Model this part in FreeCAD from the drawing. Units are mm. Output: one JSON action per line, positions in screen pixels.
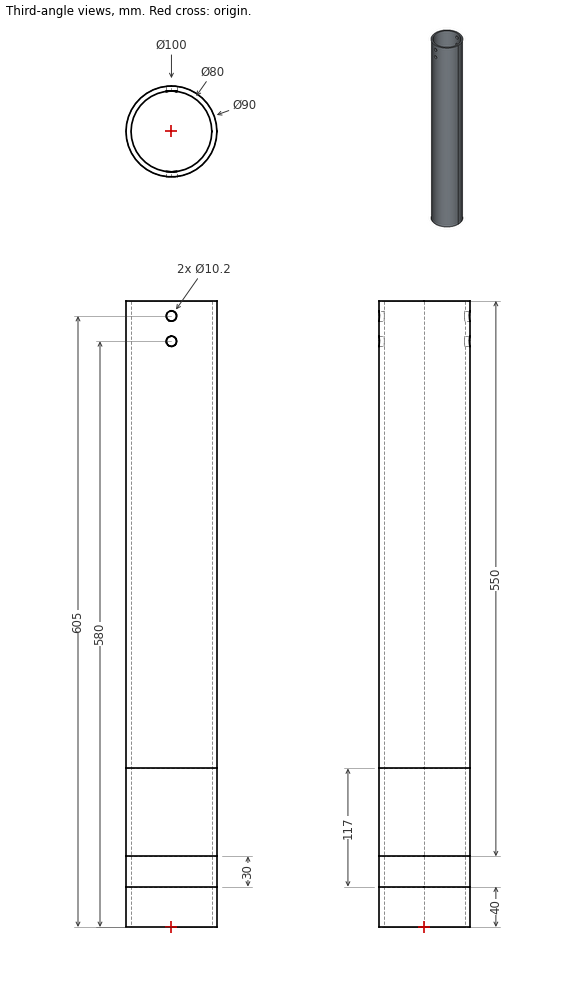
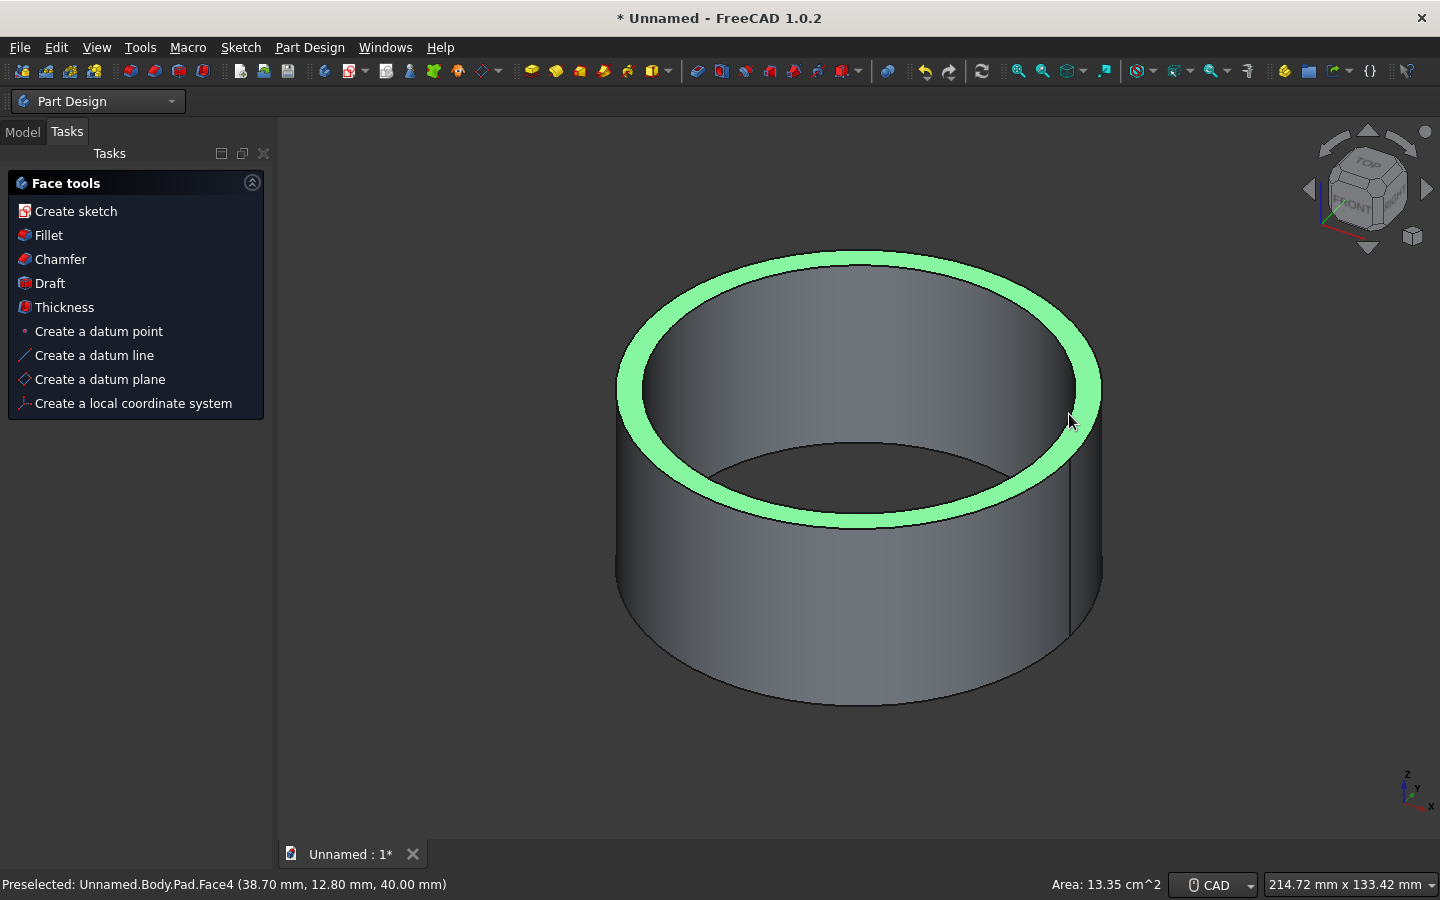
{"action": "left_click", "coordinate": [350, 72]}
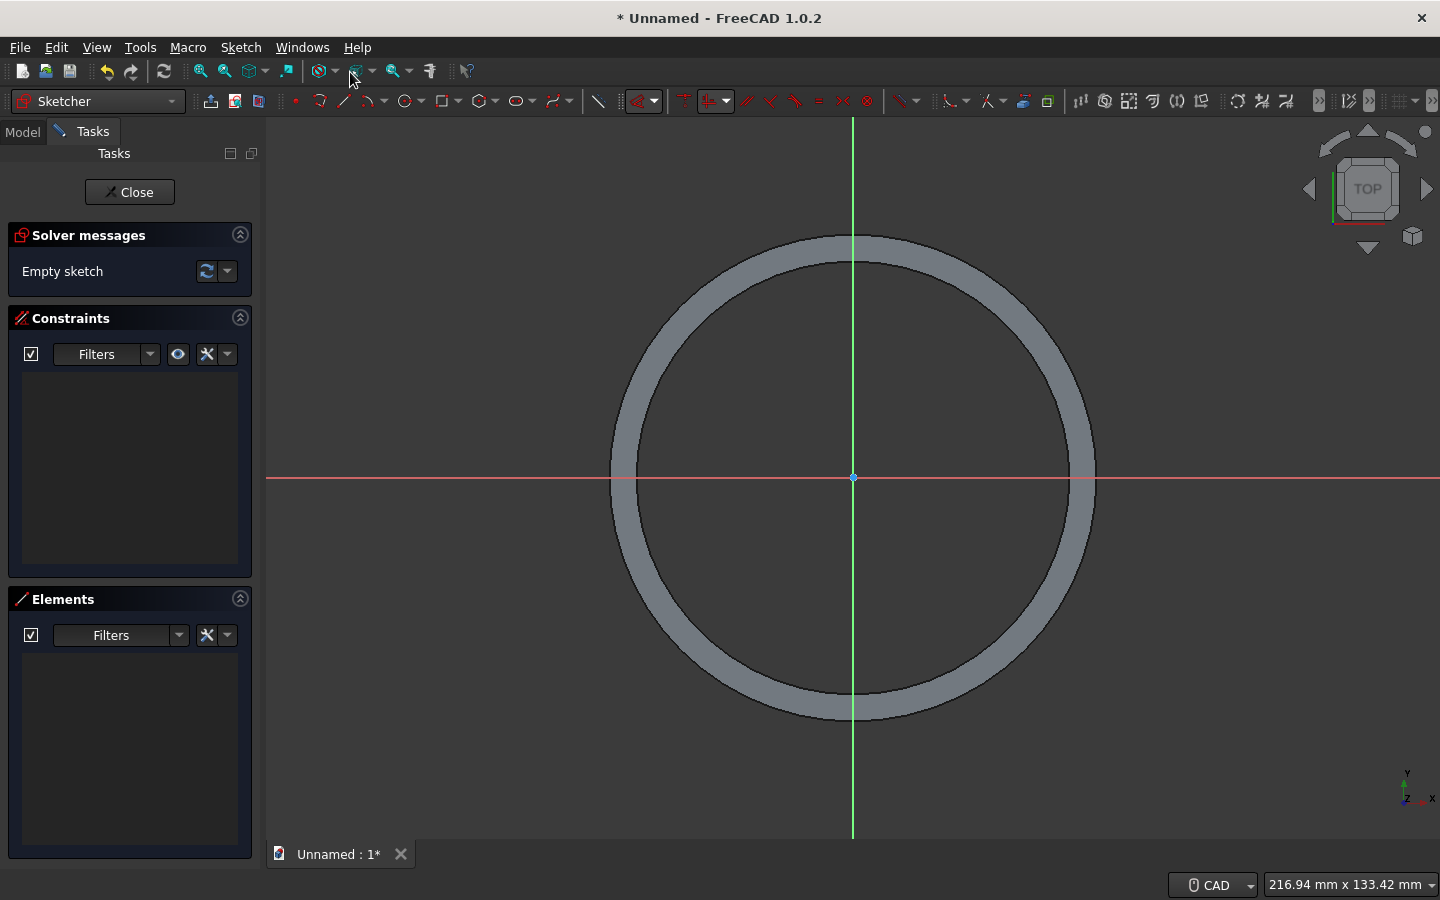
{"action": "key", "text": "g c"}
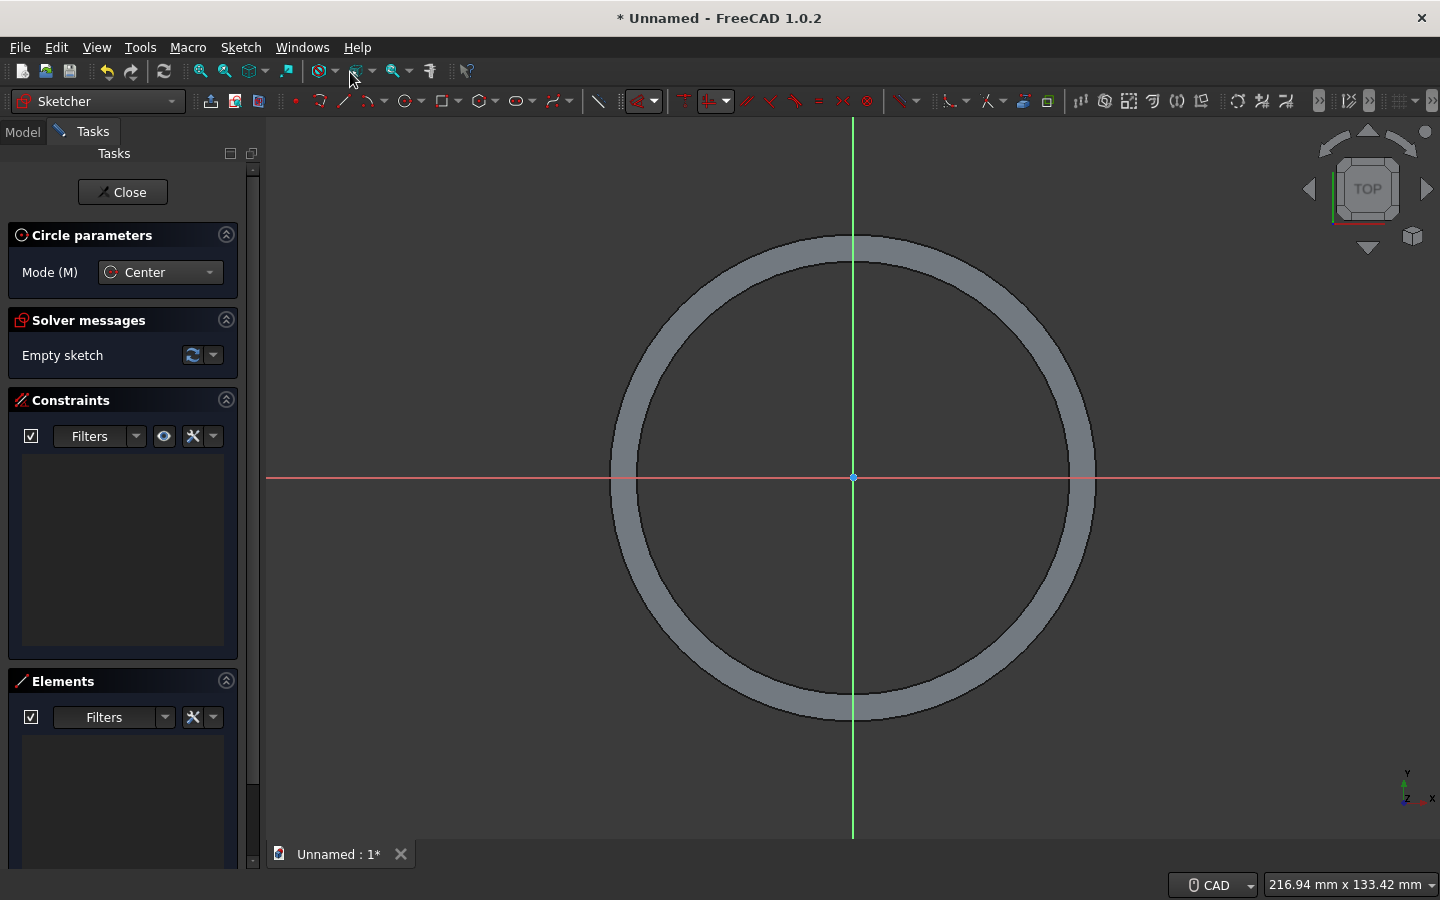
{"action": "left_click", "coordinate": [853, 478]}
{"action": "mouse_move", "coordinate": [1044, 287]}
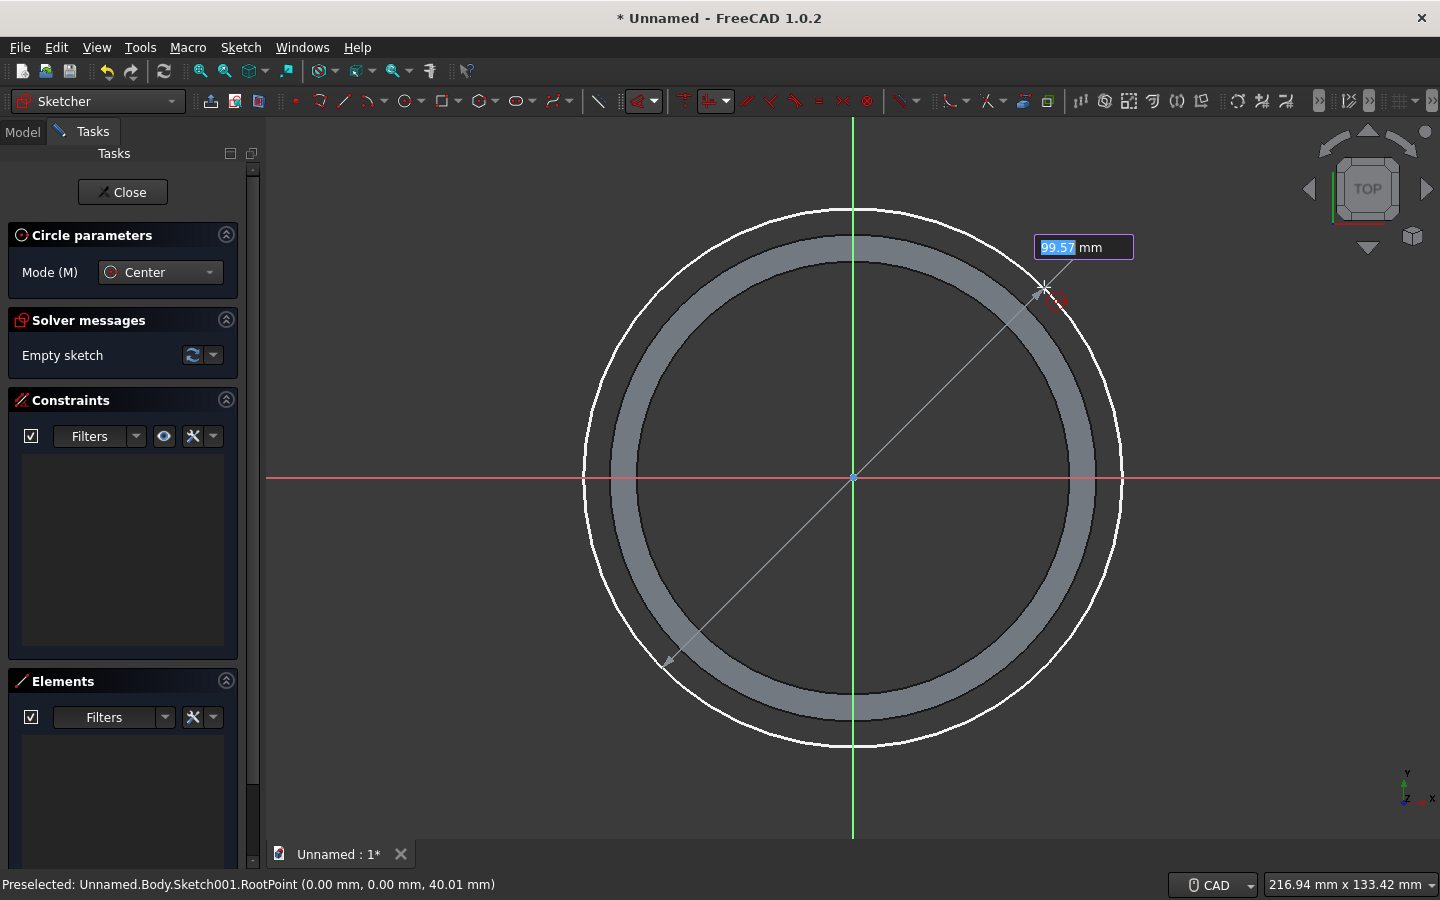
{"action": "type", "text": "100"}
{"action": "key", "text": "Return"}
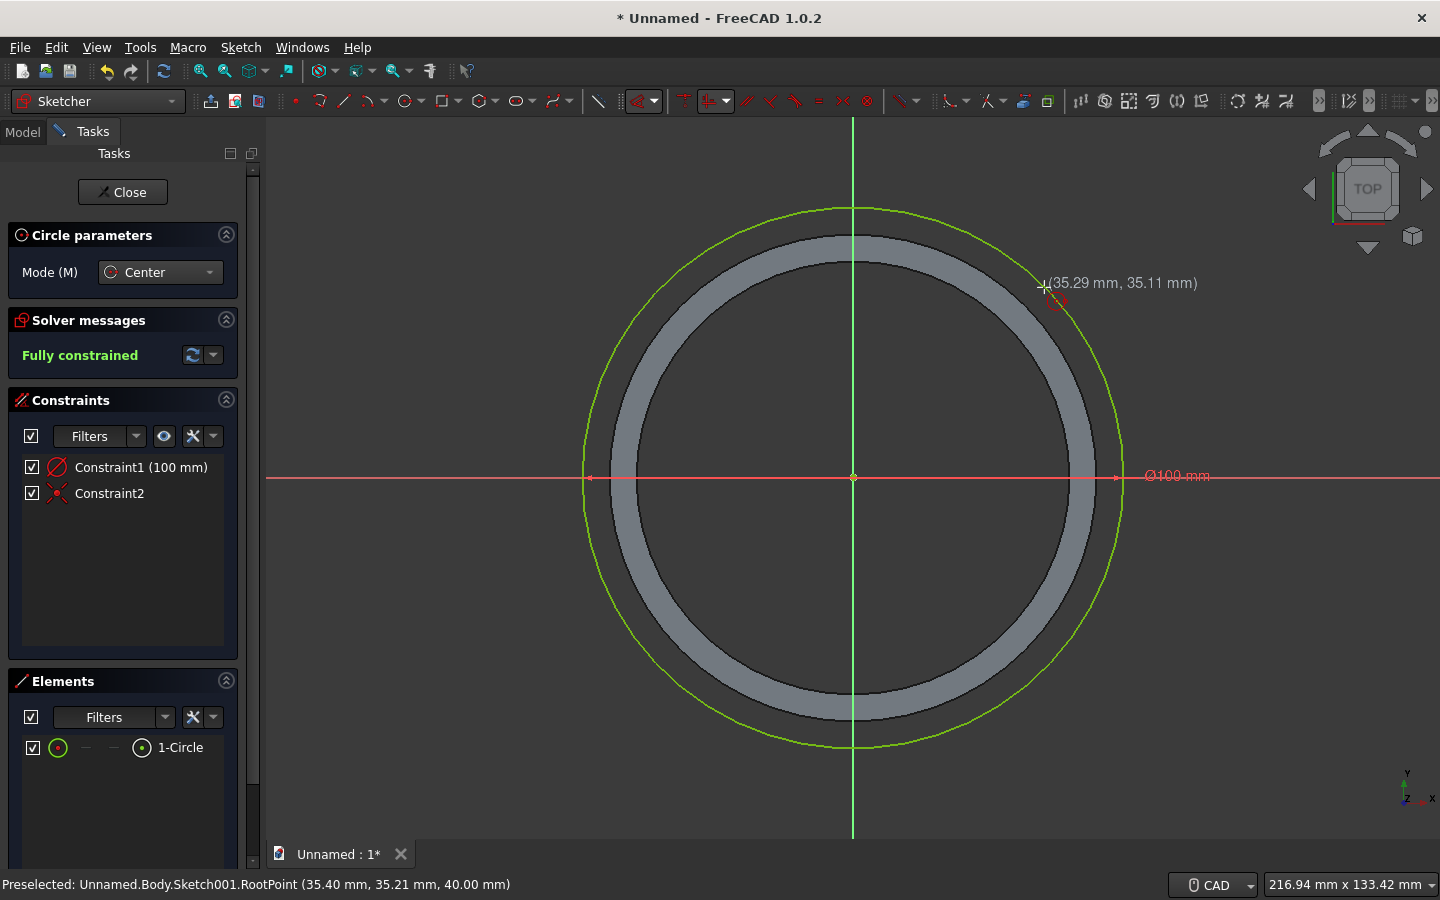
{"action": "left_click", "coordinate": [853, 478]}
{"action": "mouse_move", "coordinate": [1006, 325]}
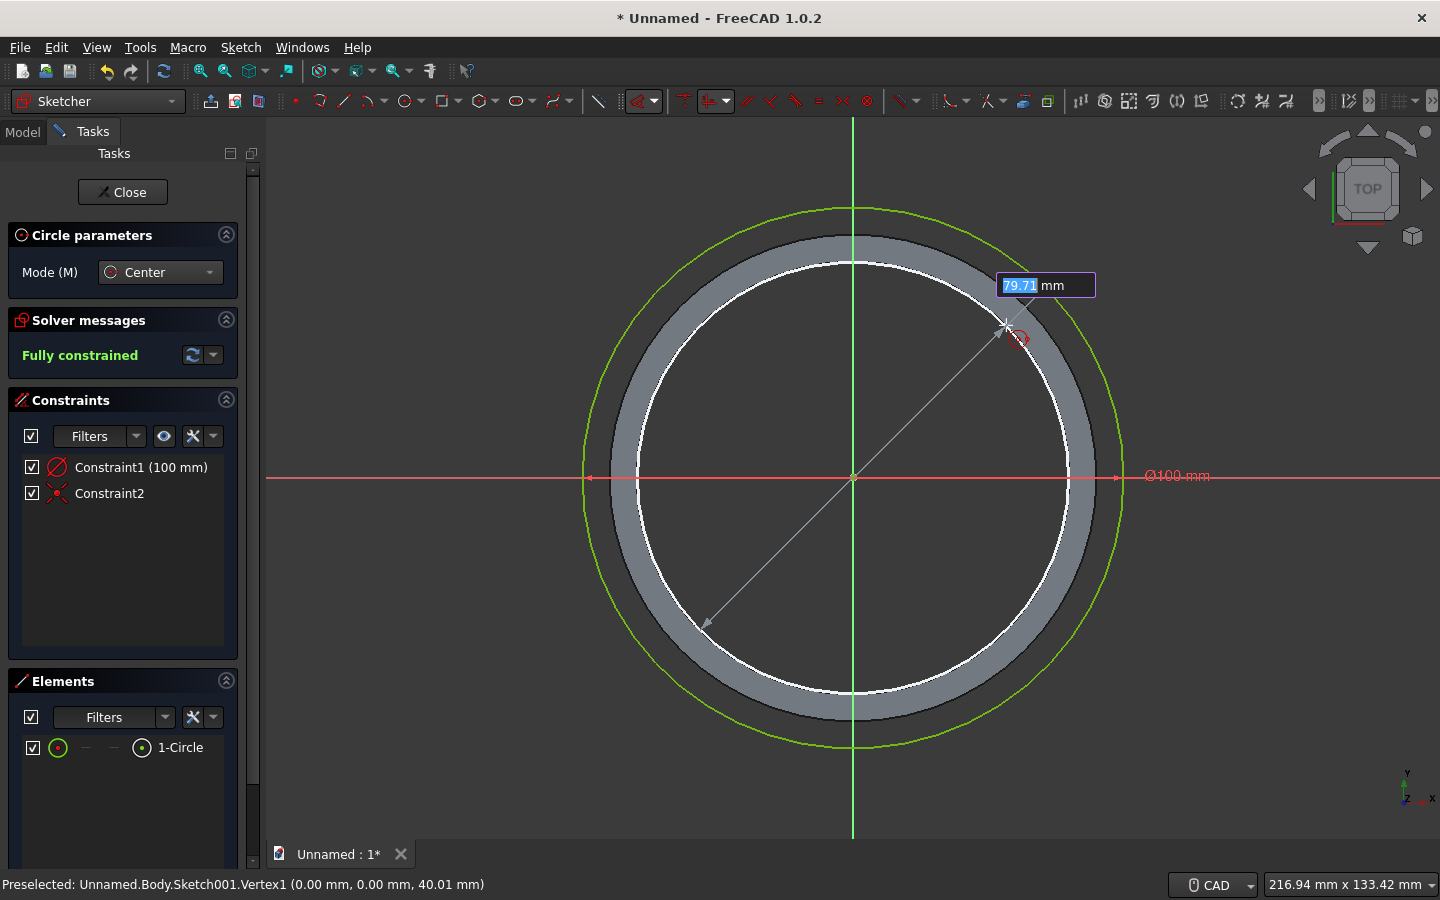
{"action": "type", "text": "80"}
{"action": "key", "text": "Return"}
{"action": "key", "text": "Escape"}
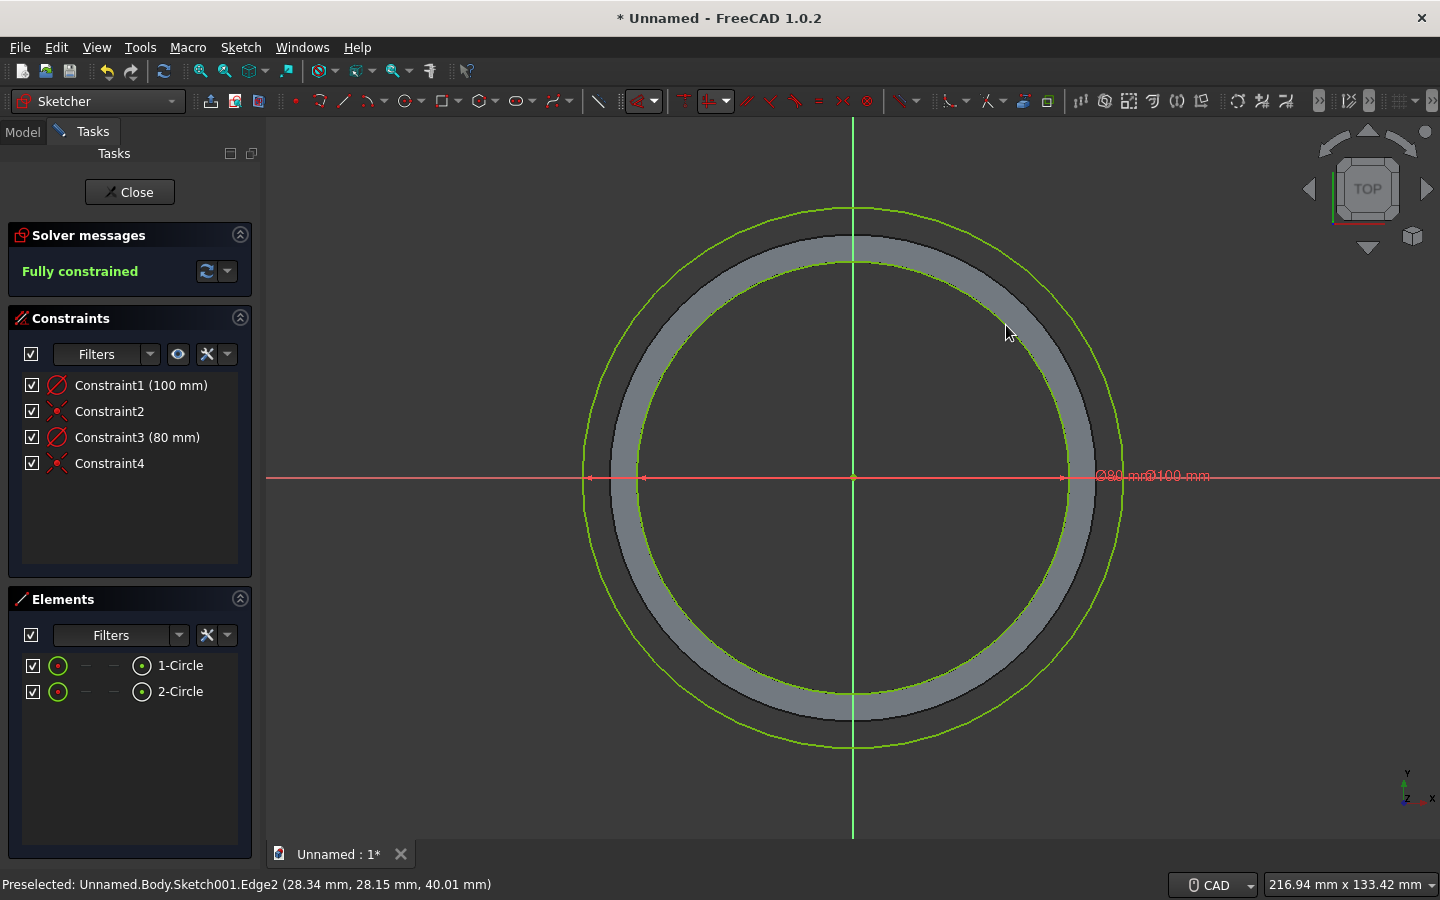
{"action": "left_click", "coordinate": [130, 192]}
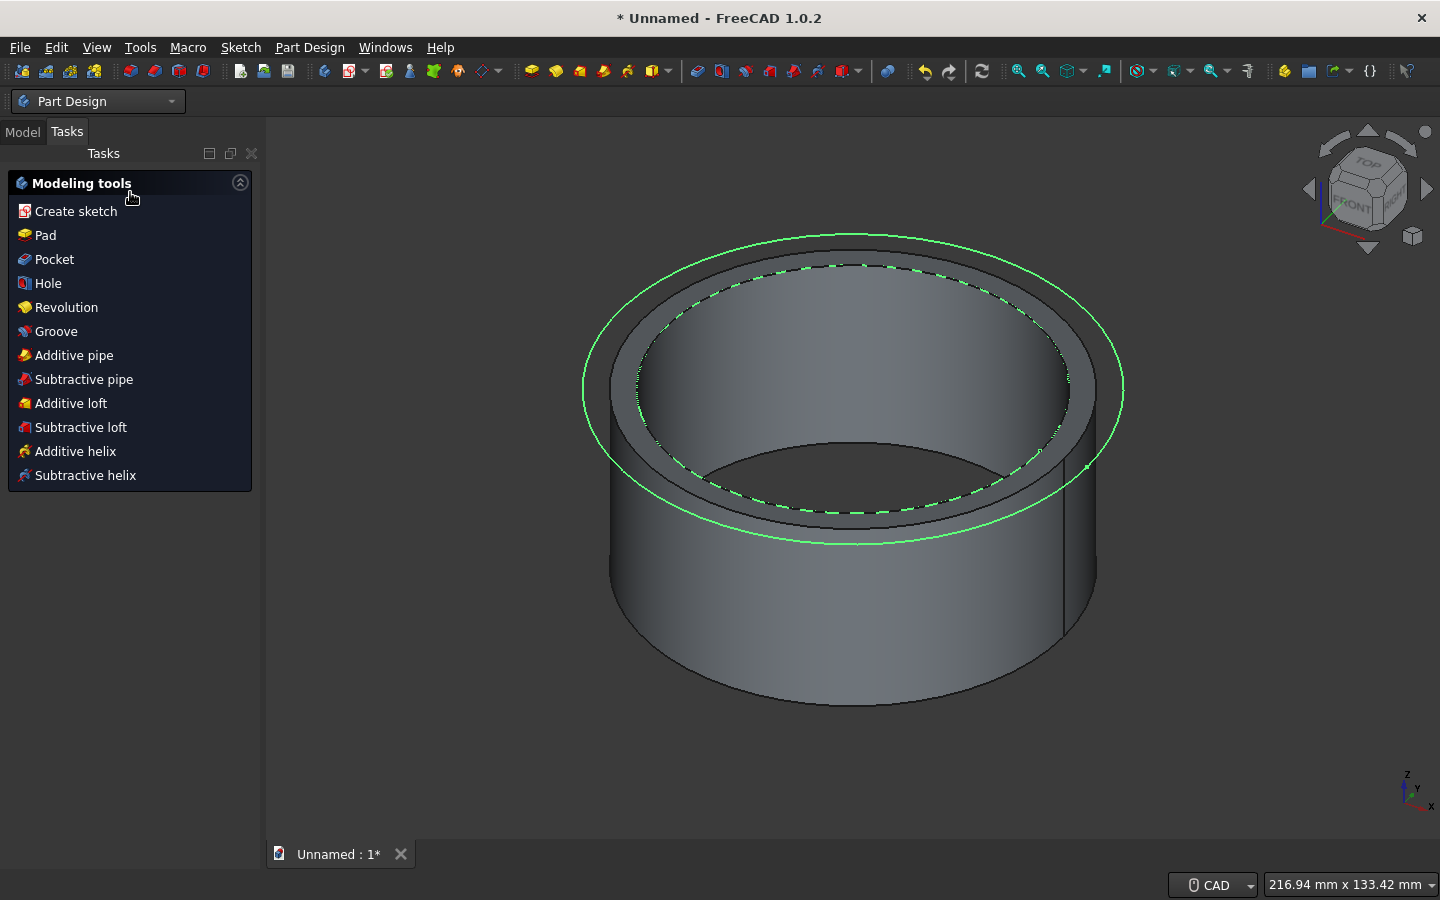
{"action": "left_click", "coordinate": [532, 72]}